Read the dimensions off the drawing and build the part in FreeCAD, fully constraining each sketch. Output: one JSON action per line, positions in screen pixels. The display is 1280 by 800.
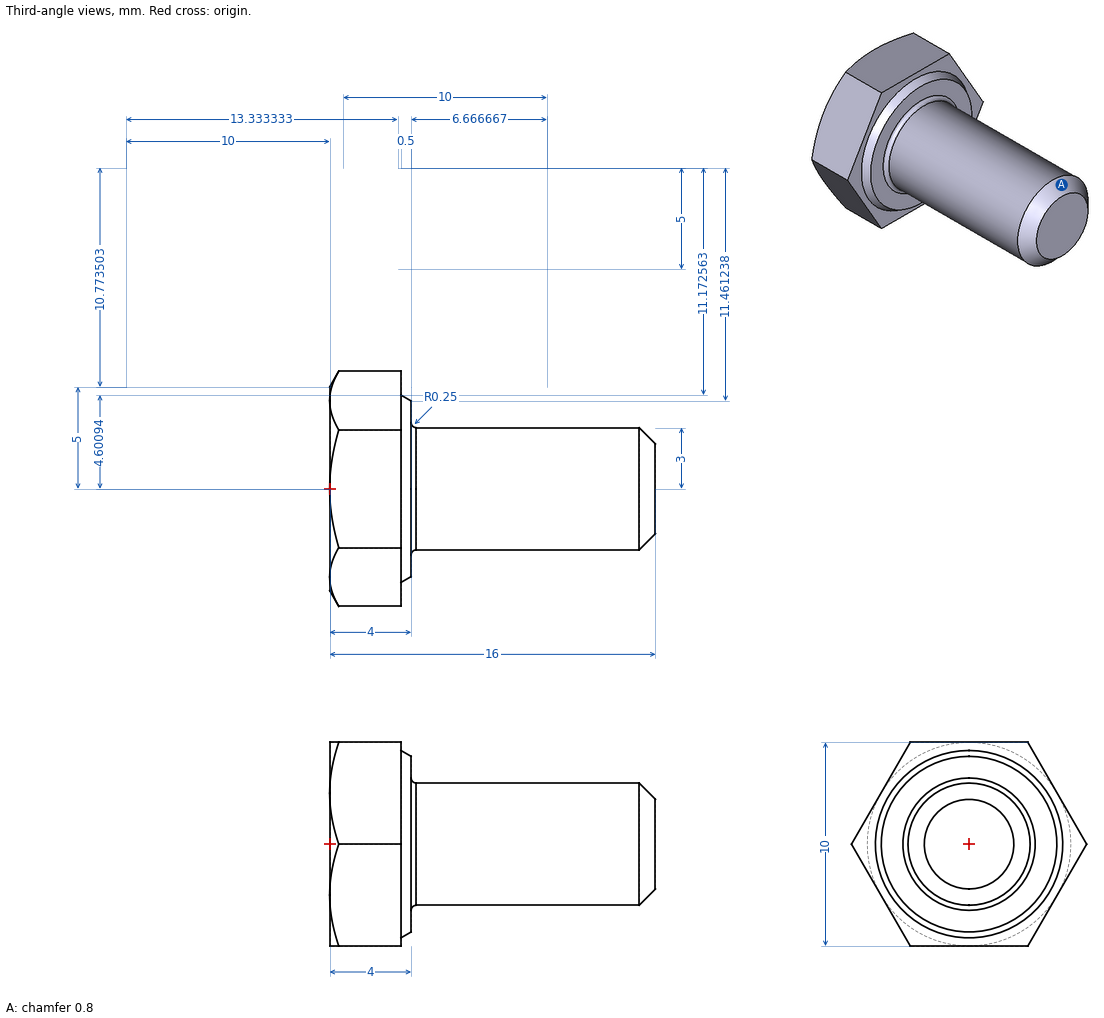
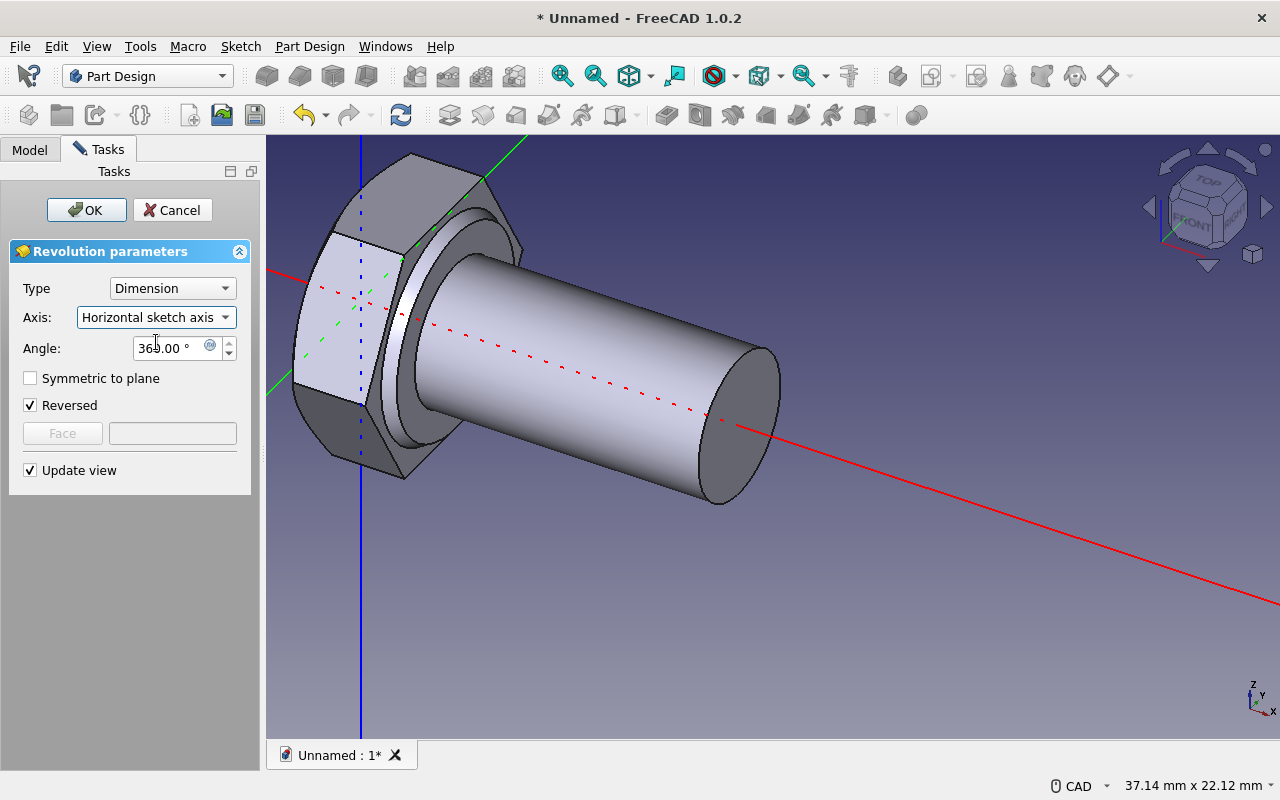
{"action": "left_click", "coordinate": [87, 210]}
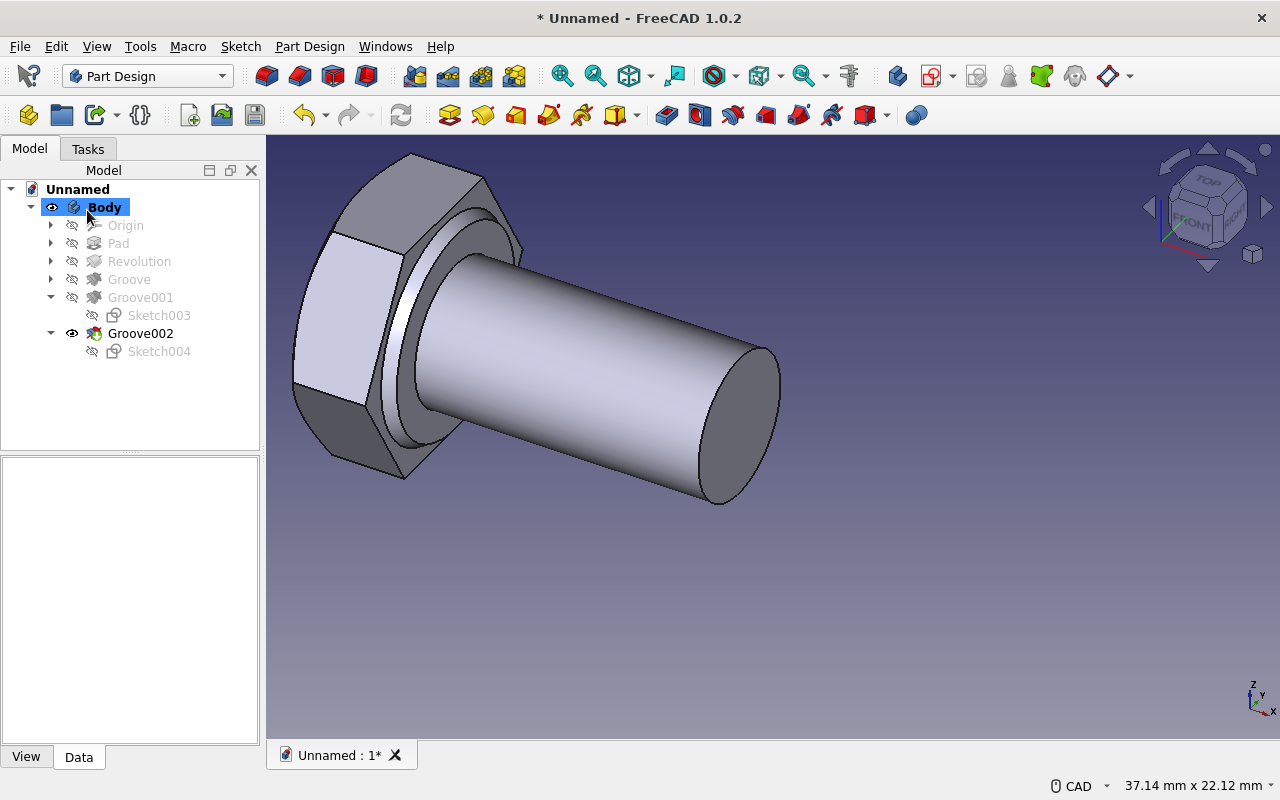
{"action": "left_click", "coordinate": [563, 76]}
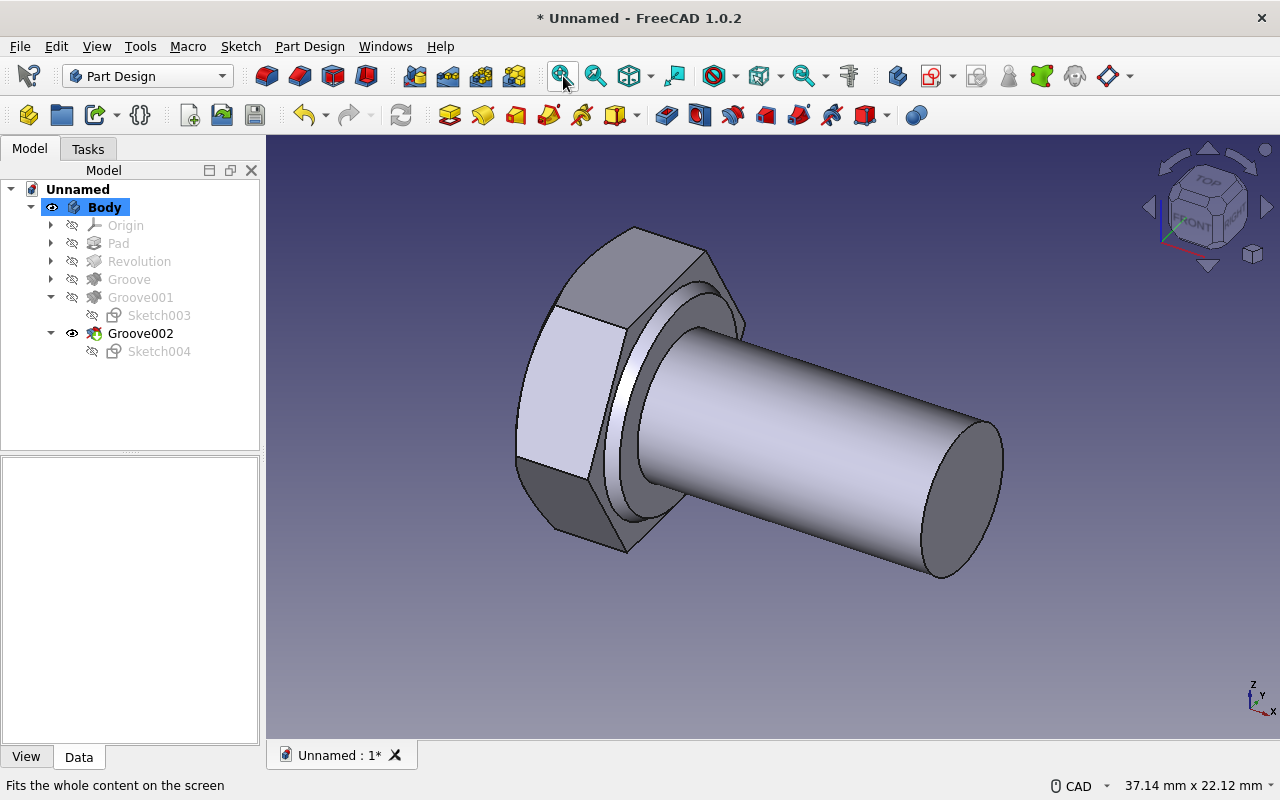
{"action": "left_click", "coordinate": [921, 539]}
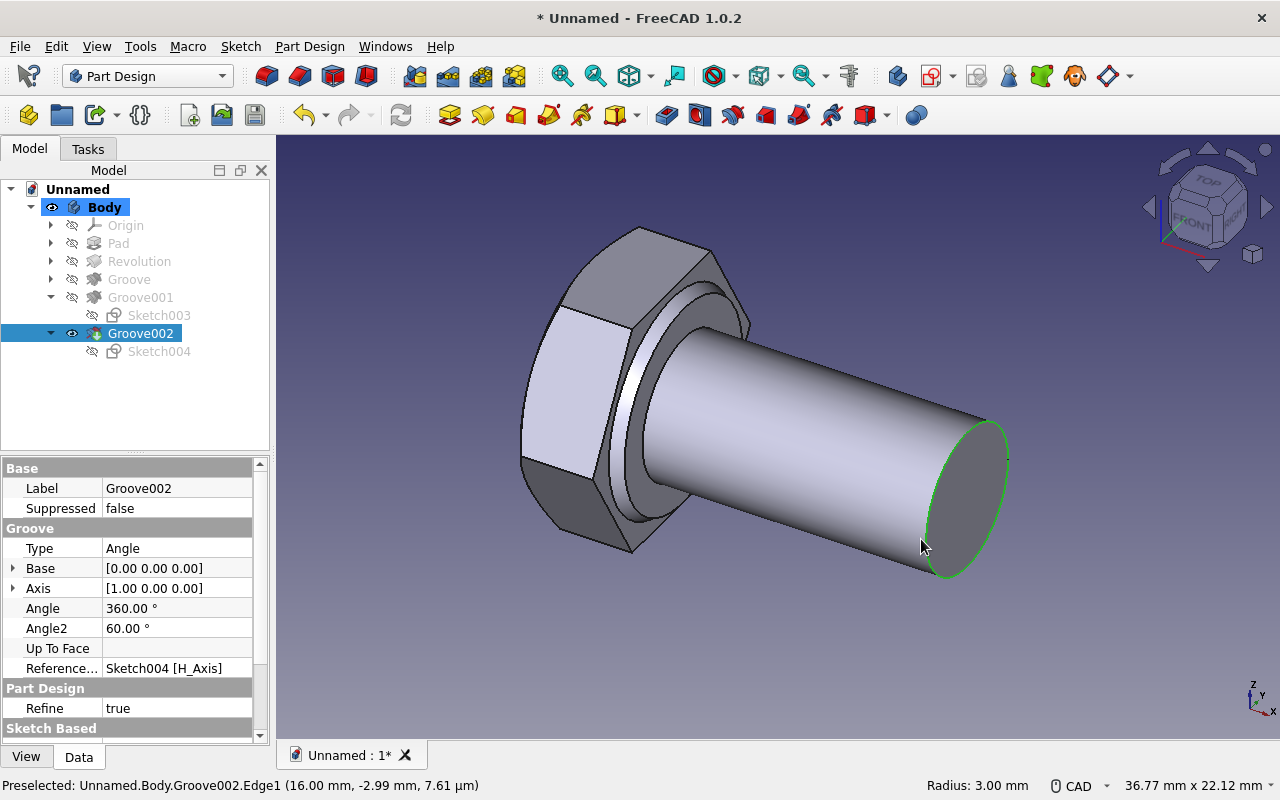
{"action": "left_click", "coordinate": [300, 76]}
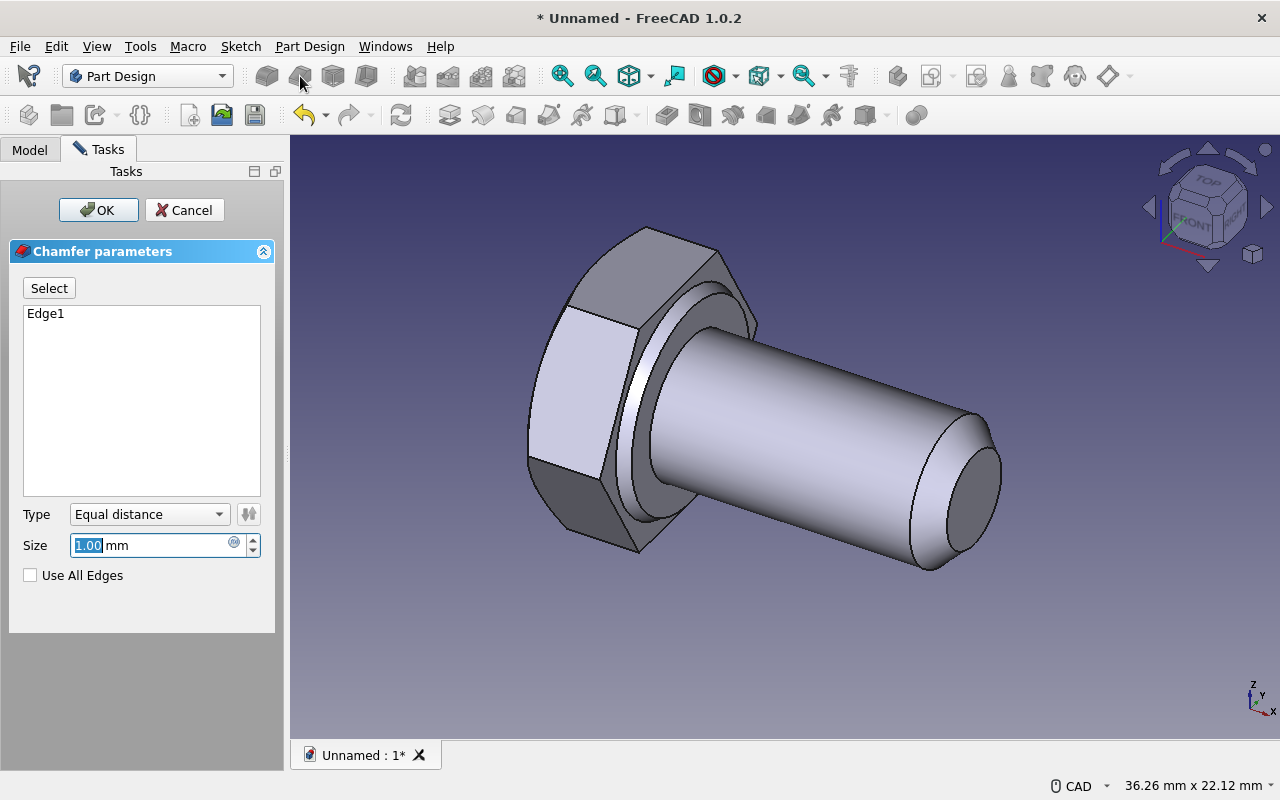
{"action": "type", "text": "0.8"}
{"action": "key", "text": "Tab"}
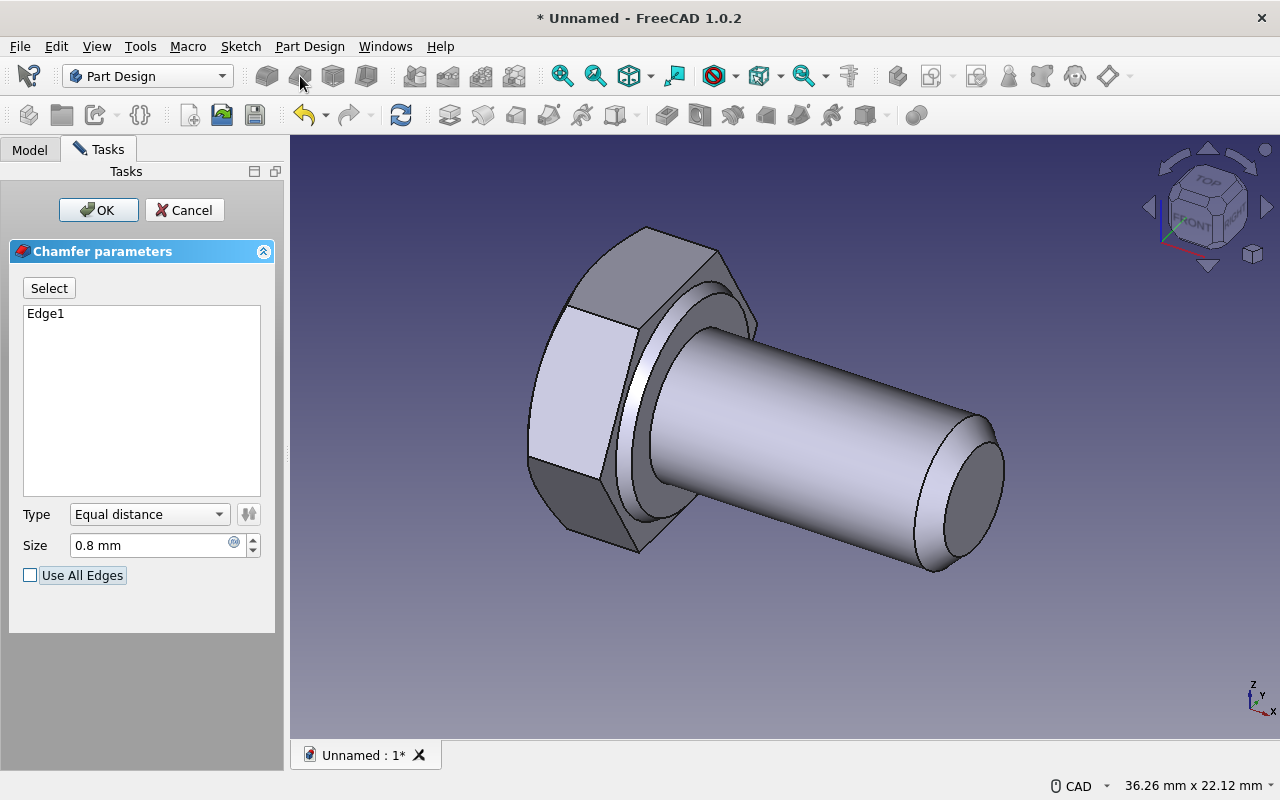
{"action": "left_click", "coordinate": [99, 210]}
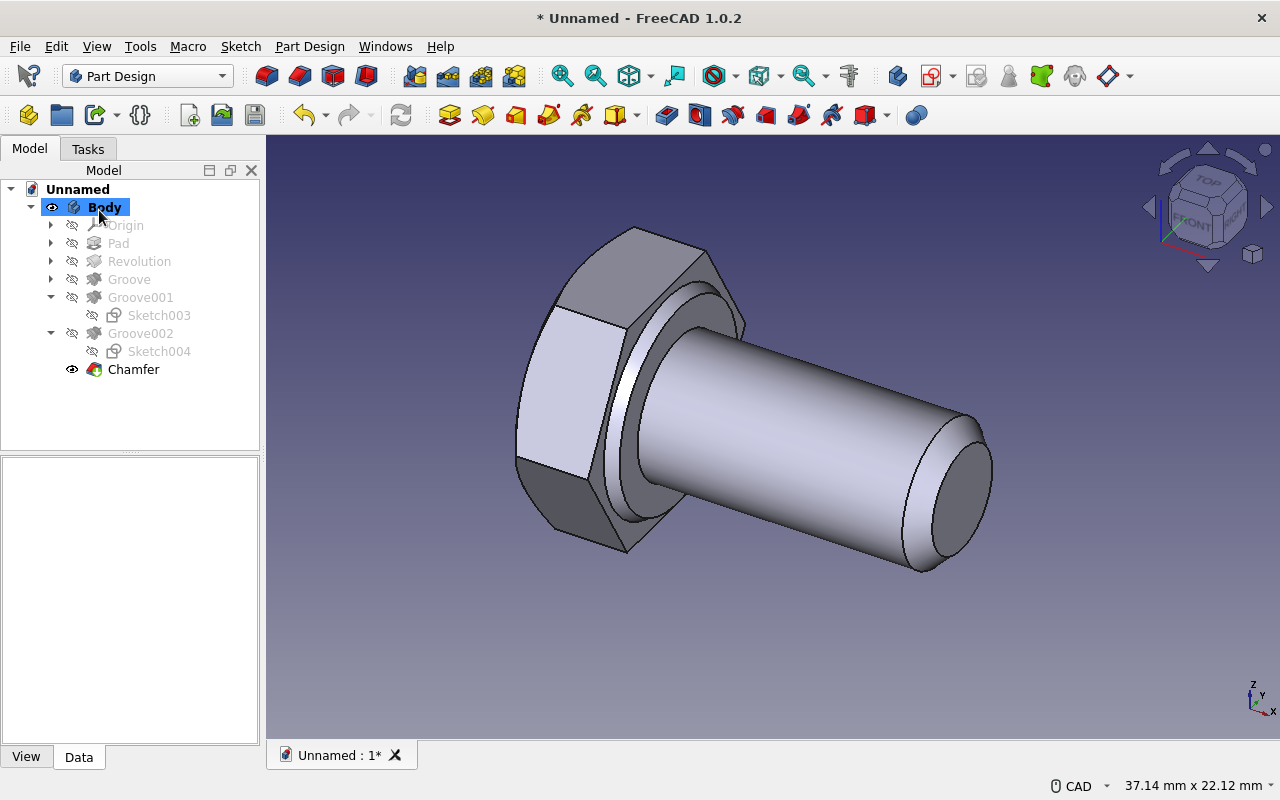
{"action": "left_click", "coordinate": [930, 76]}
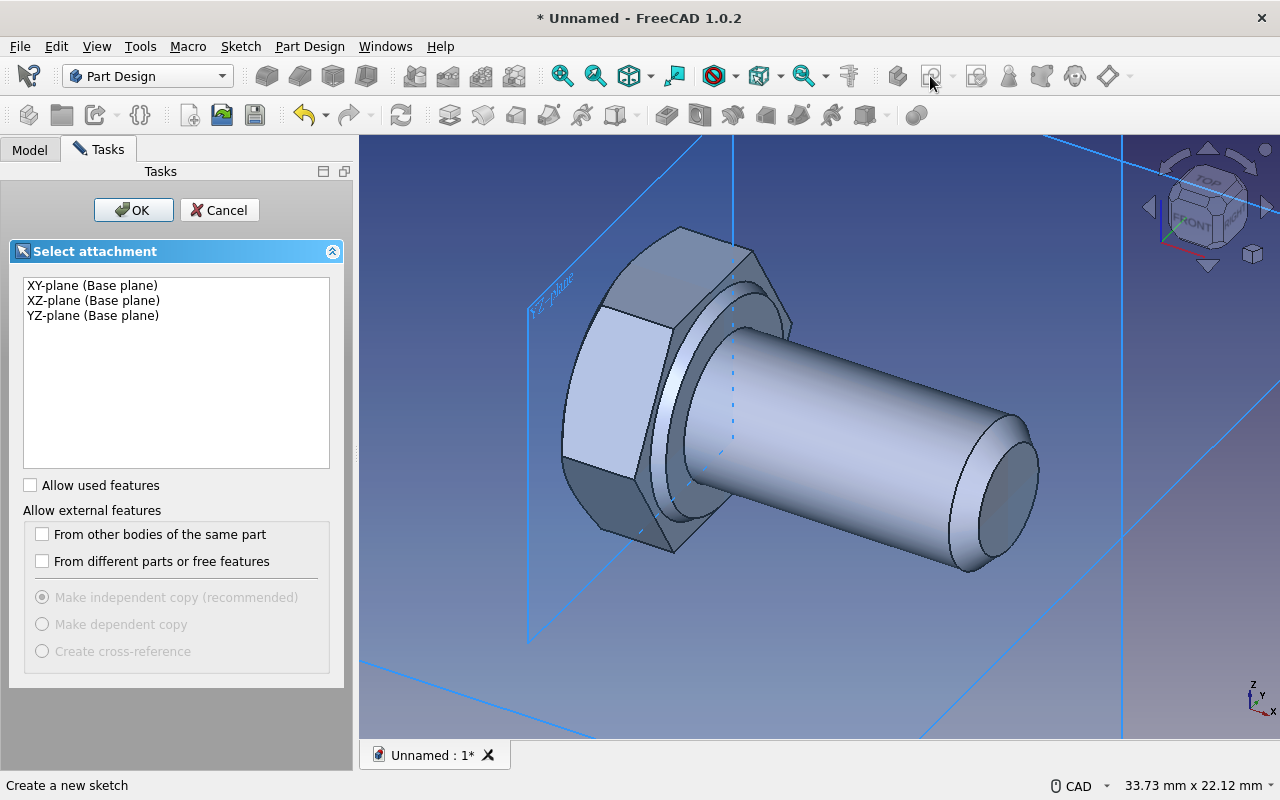
{"action": "left_click", "coordinate": [84, 286]}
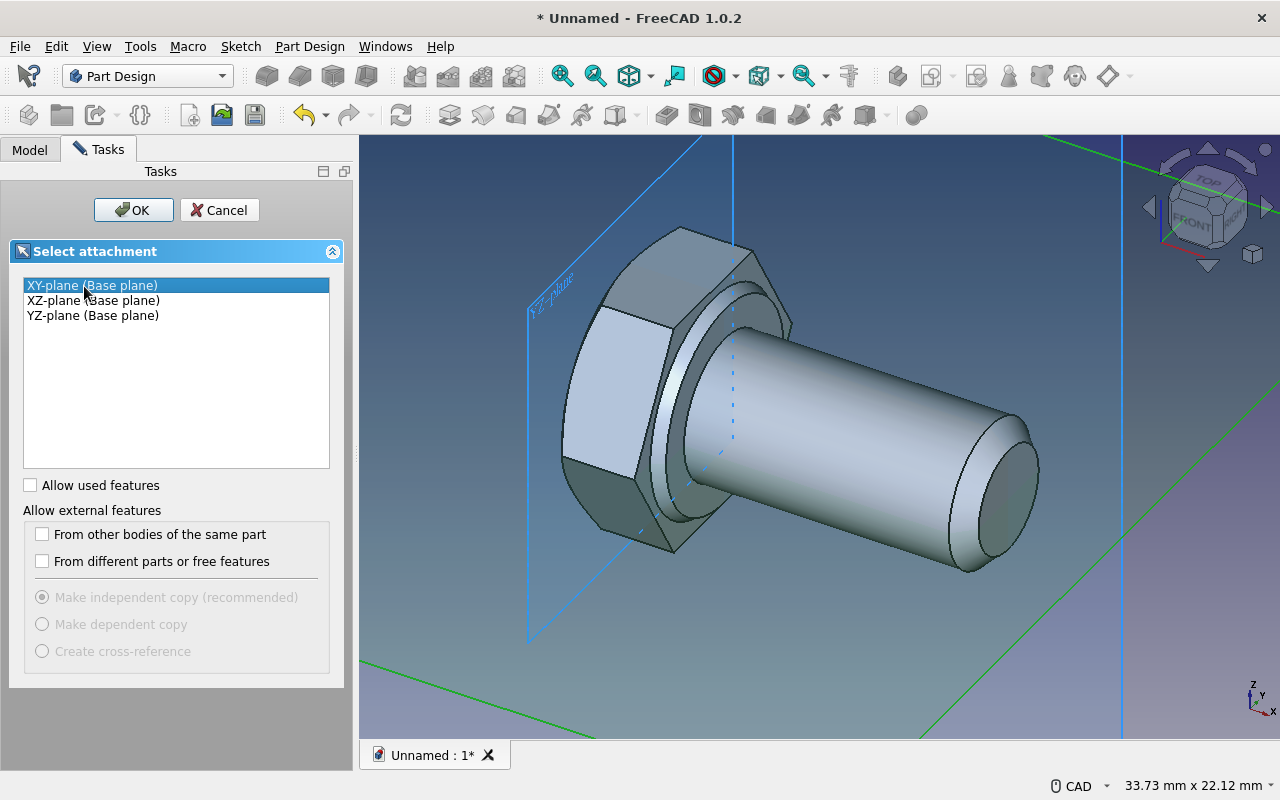
{"action": "left_click", "coordinate": [134, 210]}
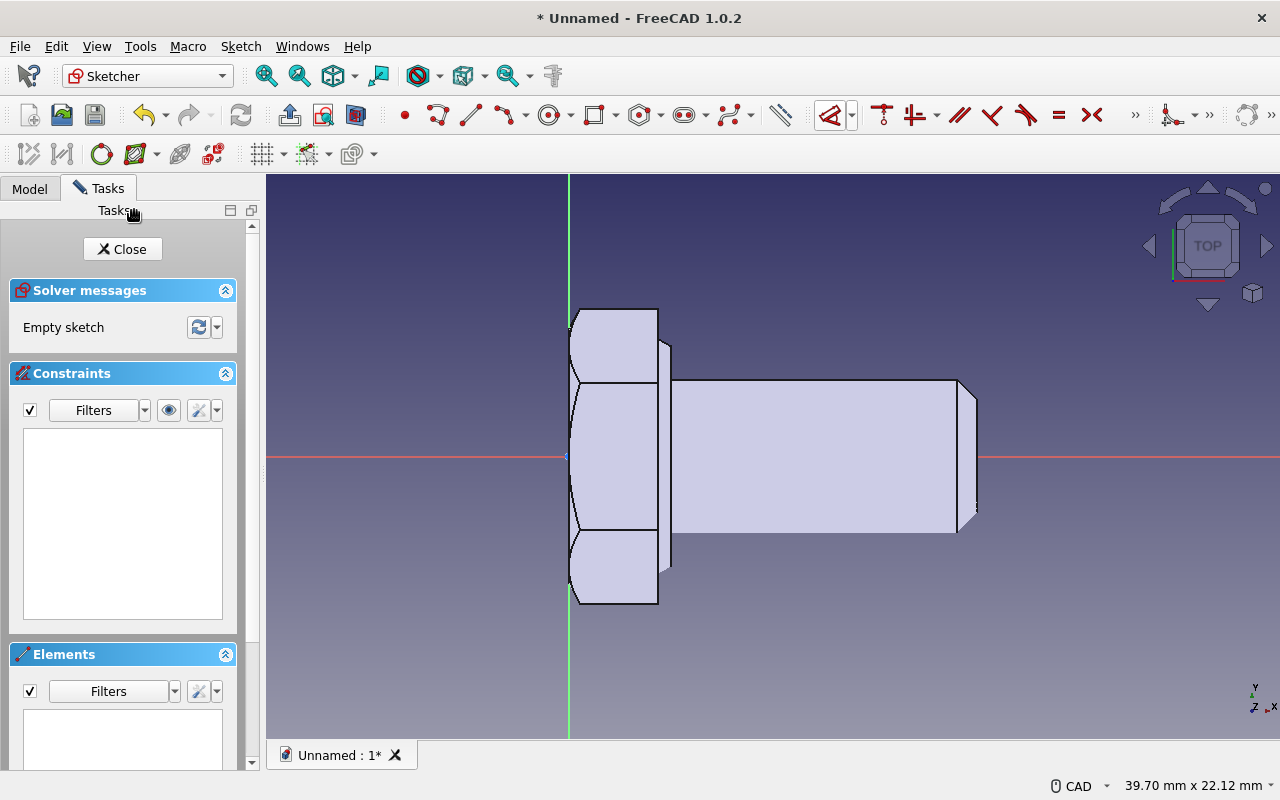
{"action": "left_click", "coordinate": [356, 116]}